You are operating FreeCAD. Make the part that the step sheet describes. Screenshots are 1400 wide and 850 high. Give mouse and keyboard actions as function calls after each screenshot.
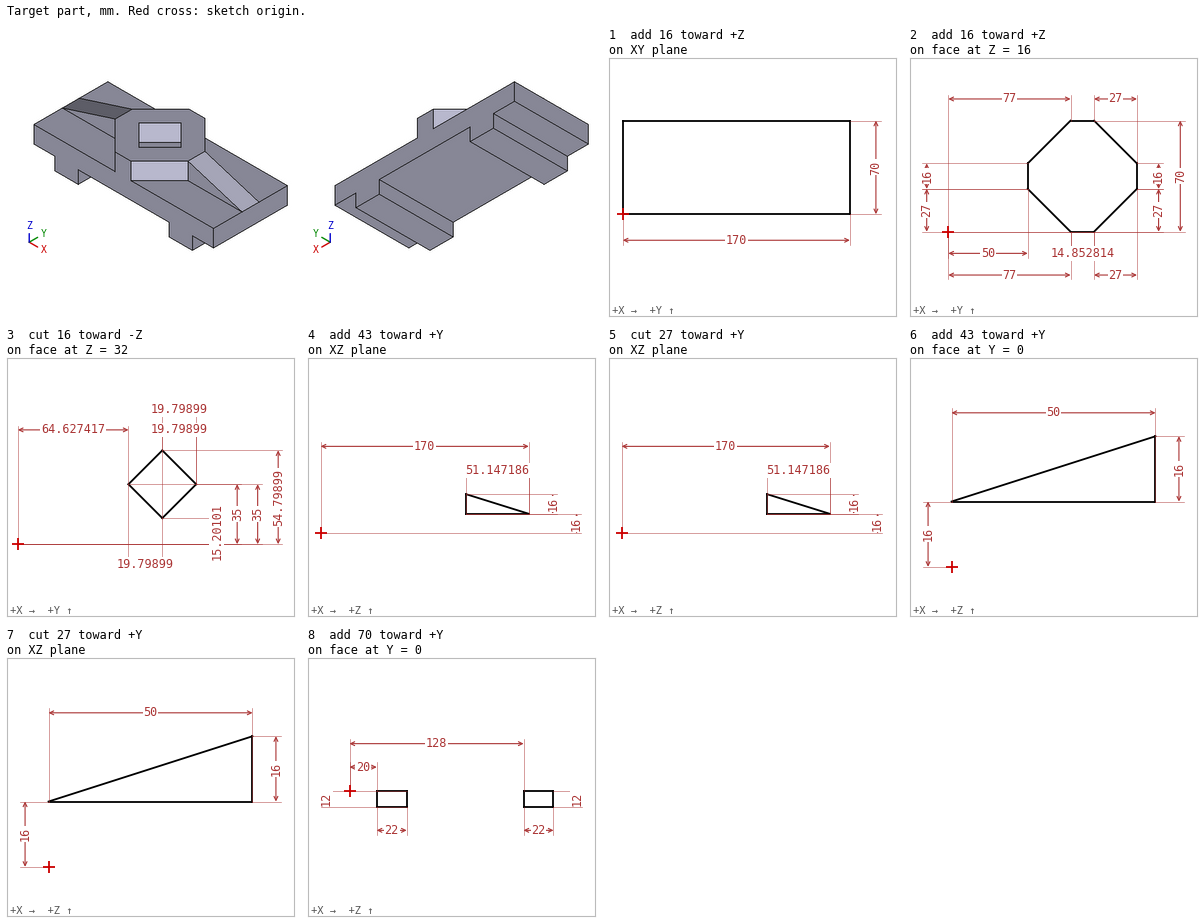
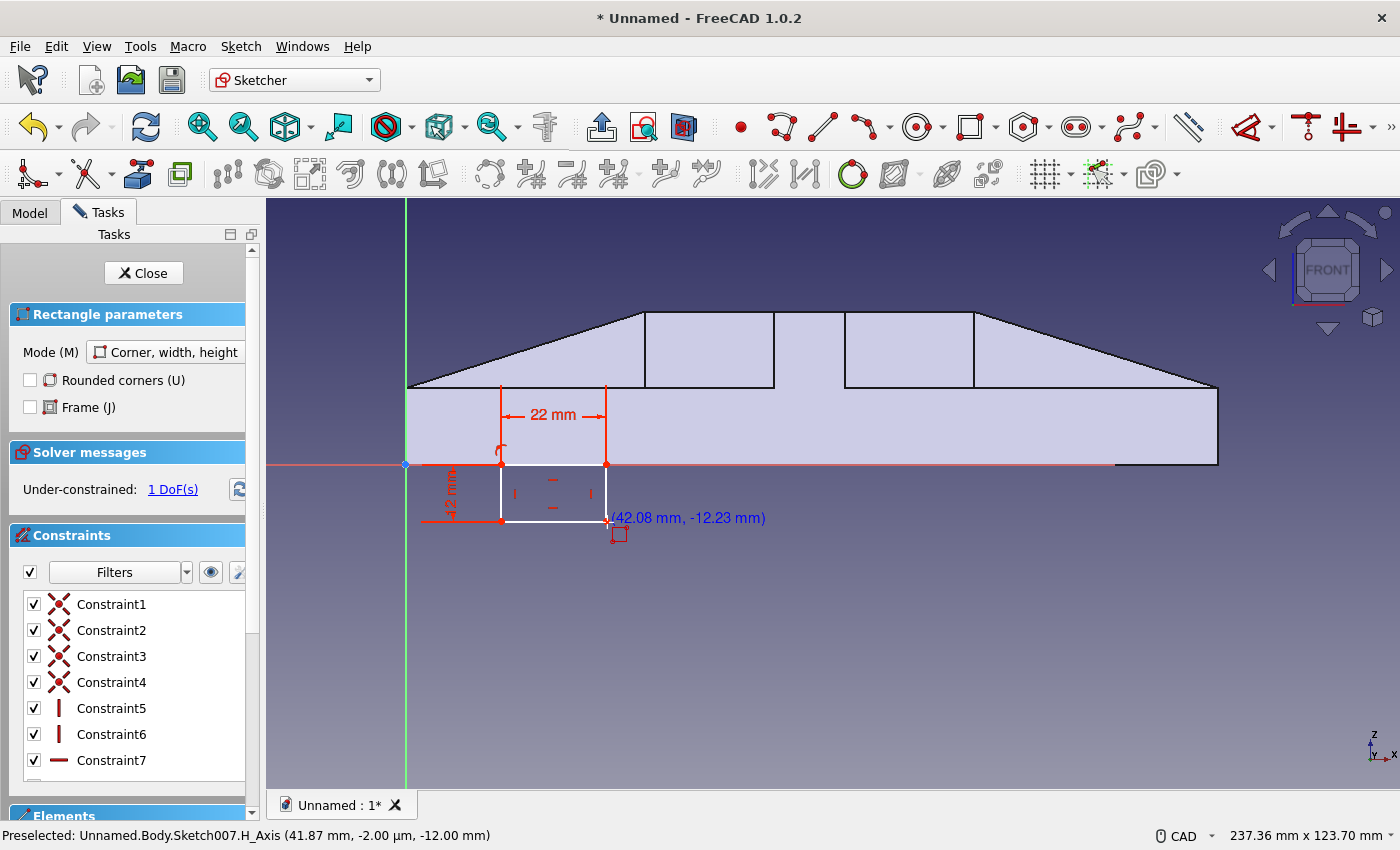
click(1017, 465)
move(1123, 522)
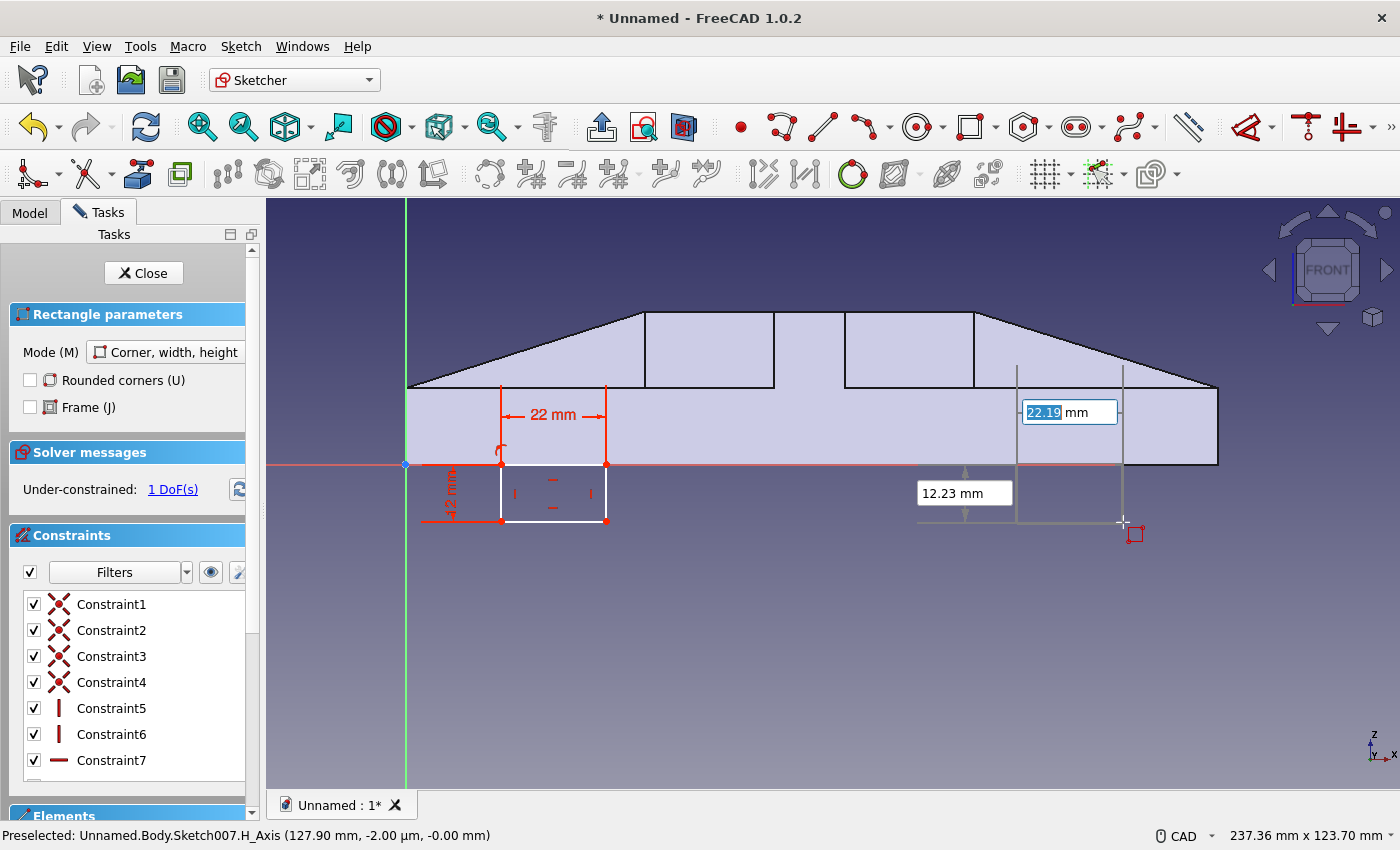
text(22)
key(Tab)
text(12)
key(Return)
key(Escape)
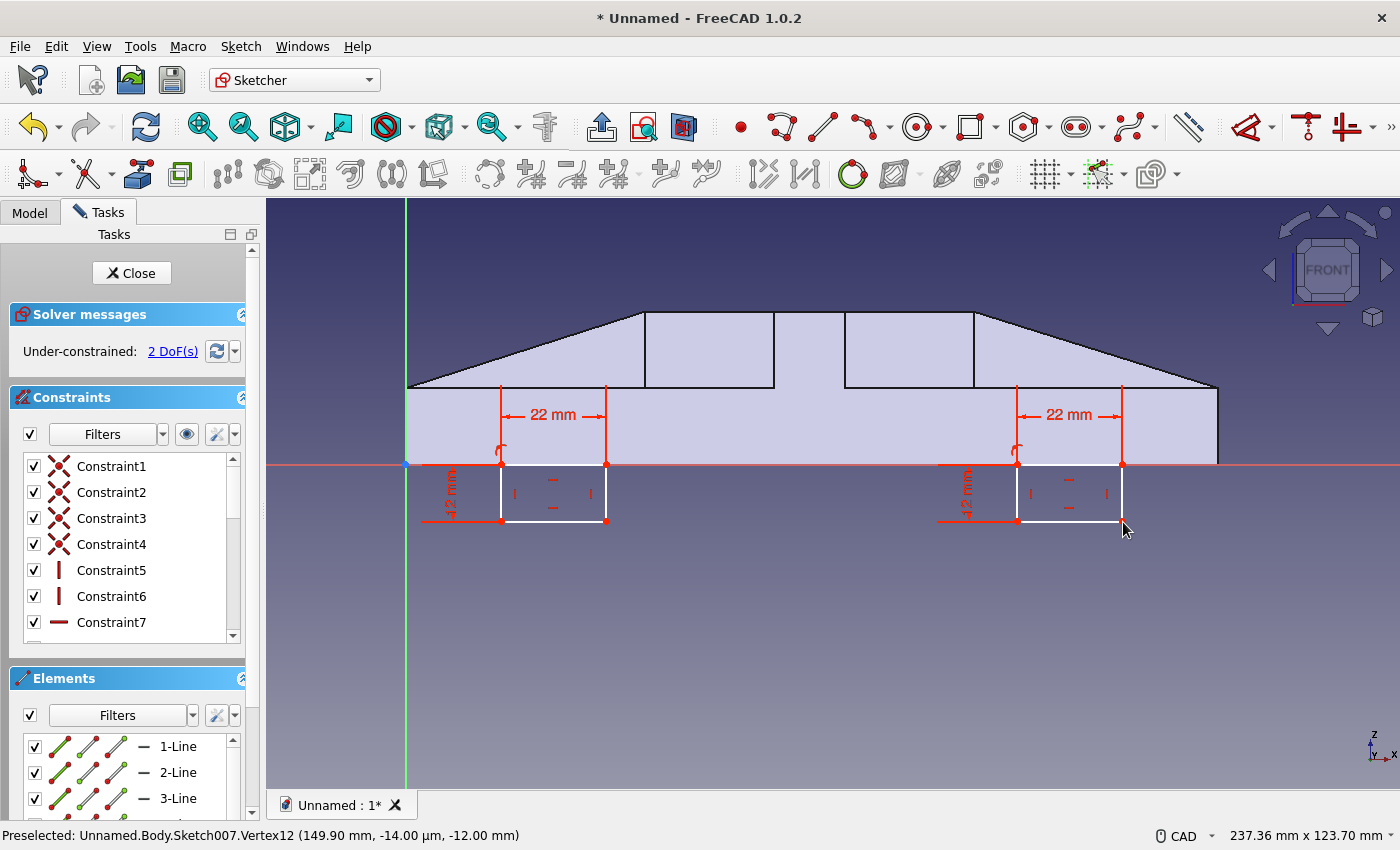
click(1246, 128)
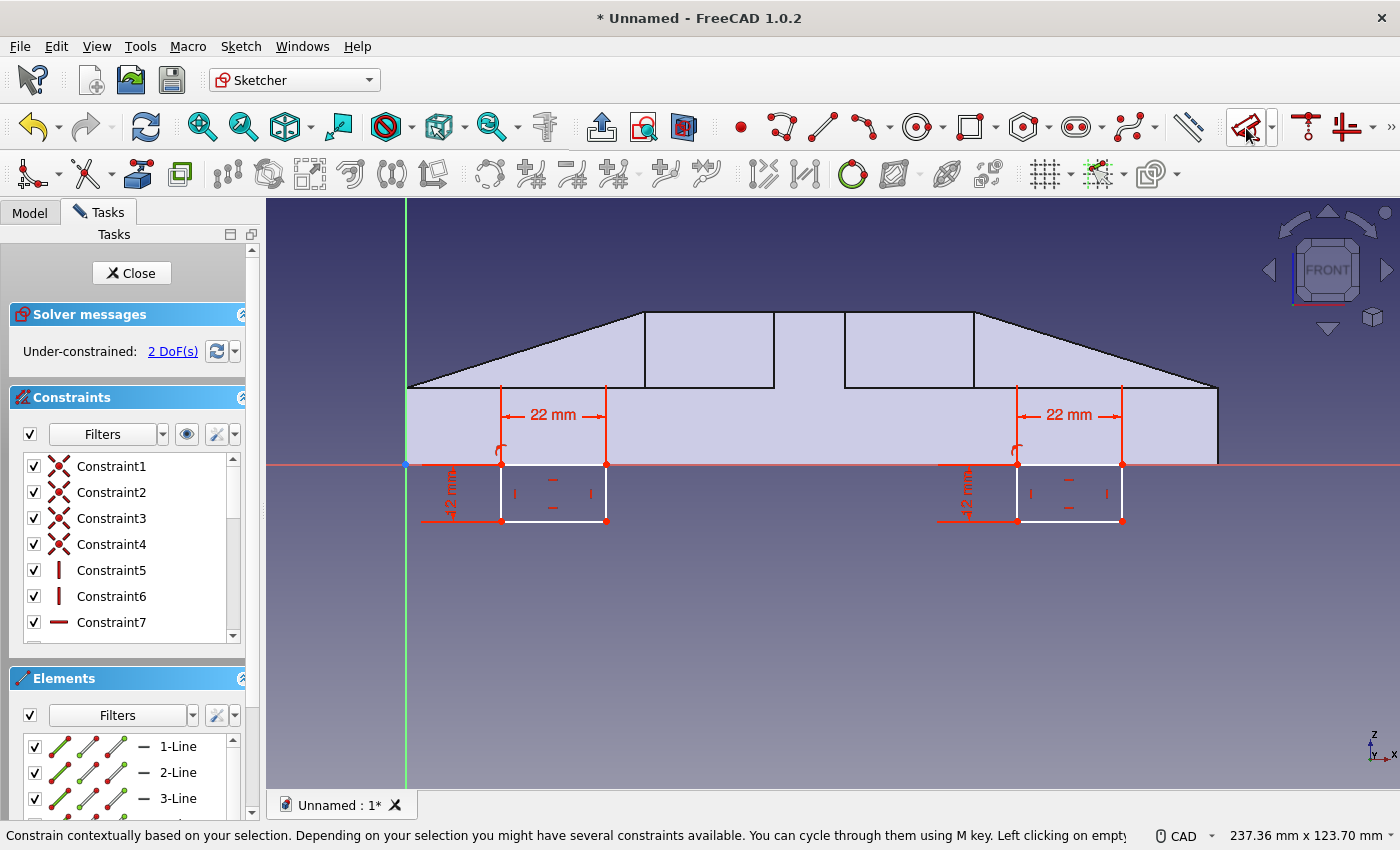
click(501, 465)
click(453, 431)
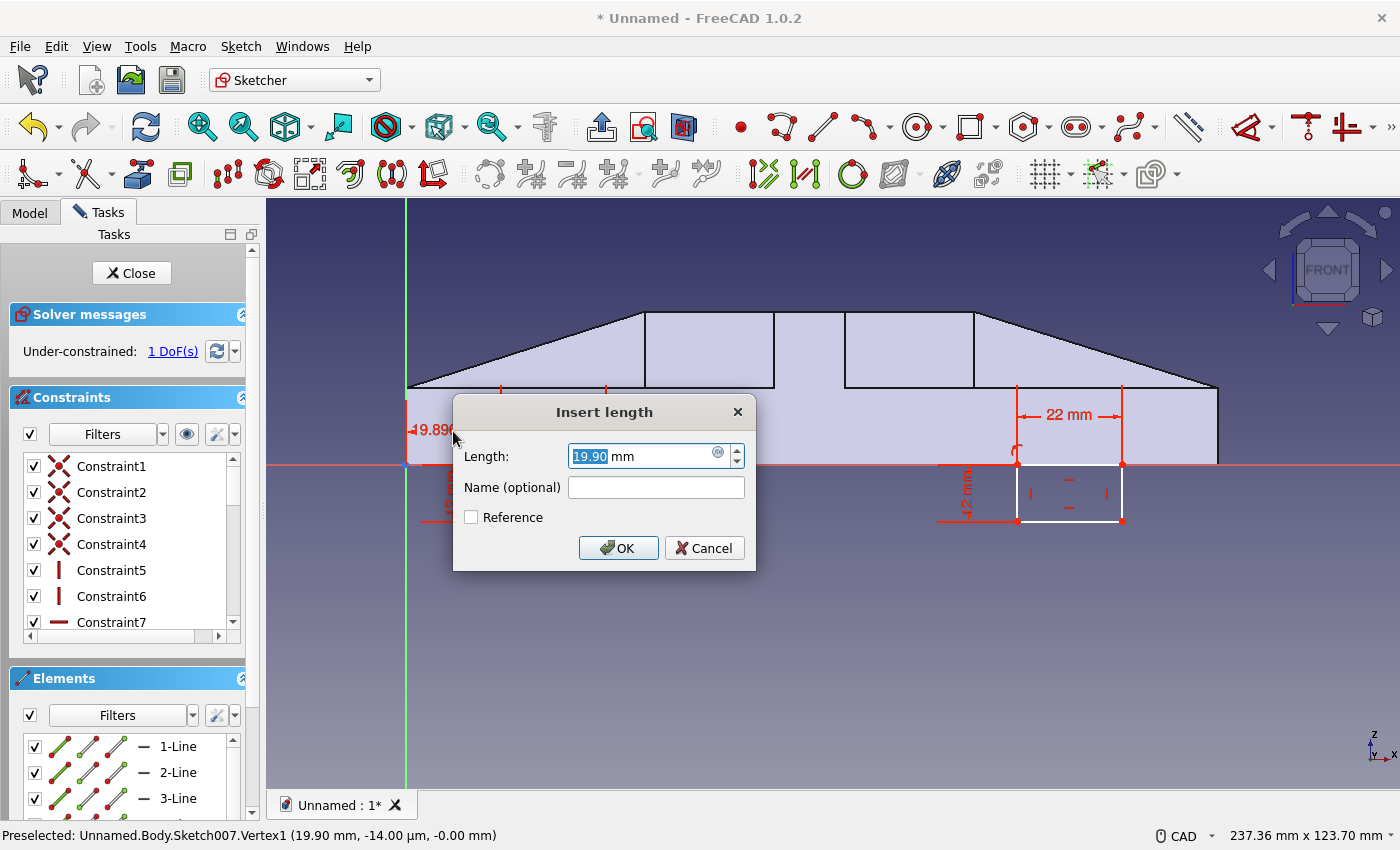
text(20)
key(Return)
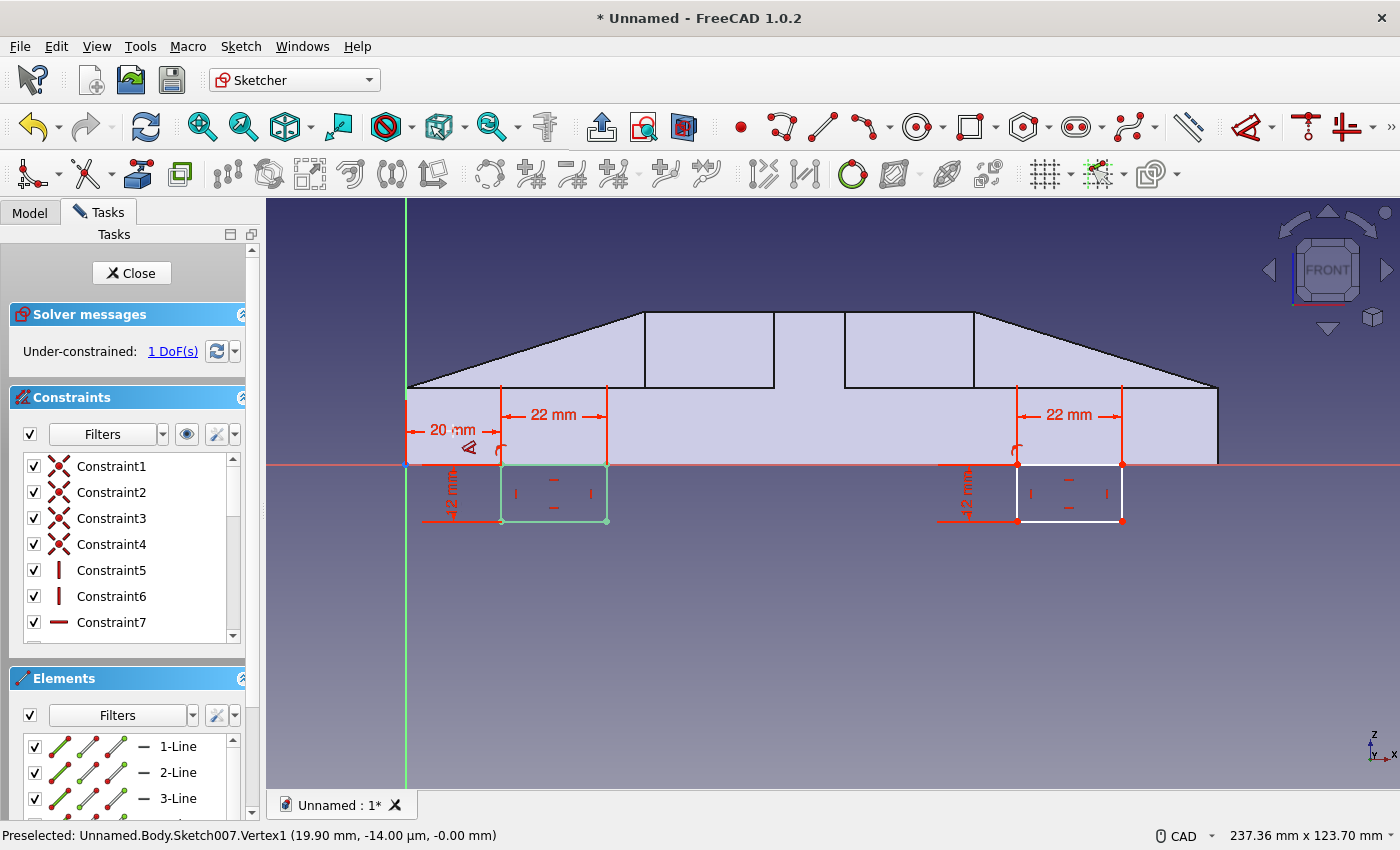
click(1017, 465)
click(711, 431)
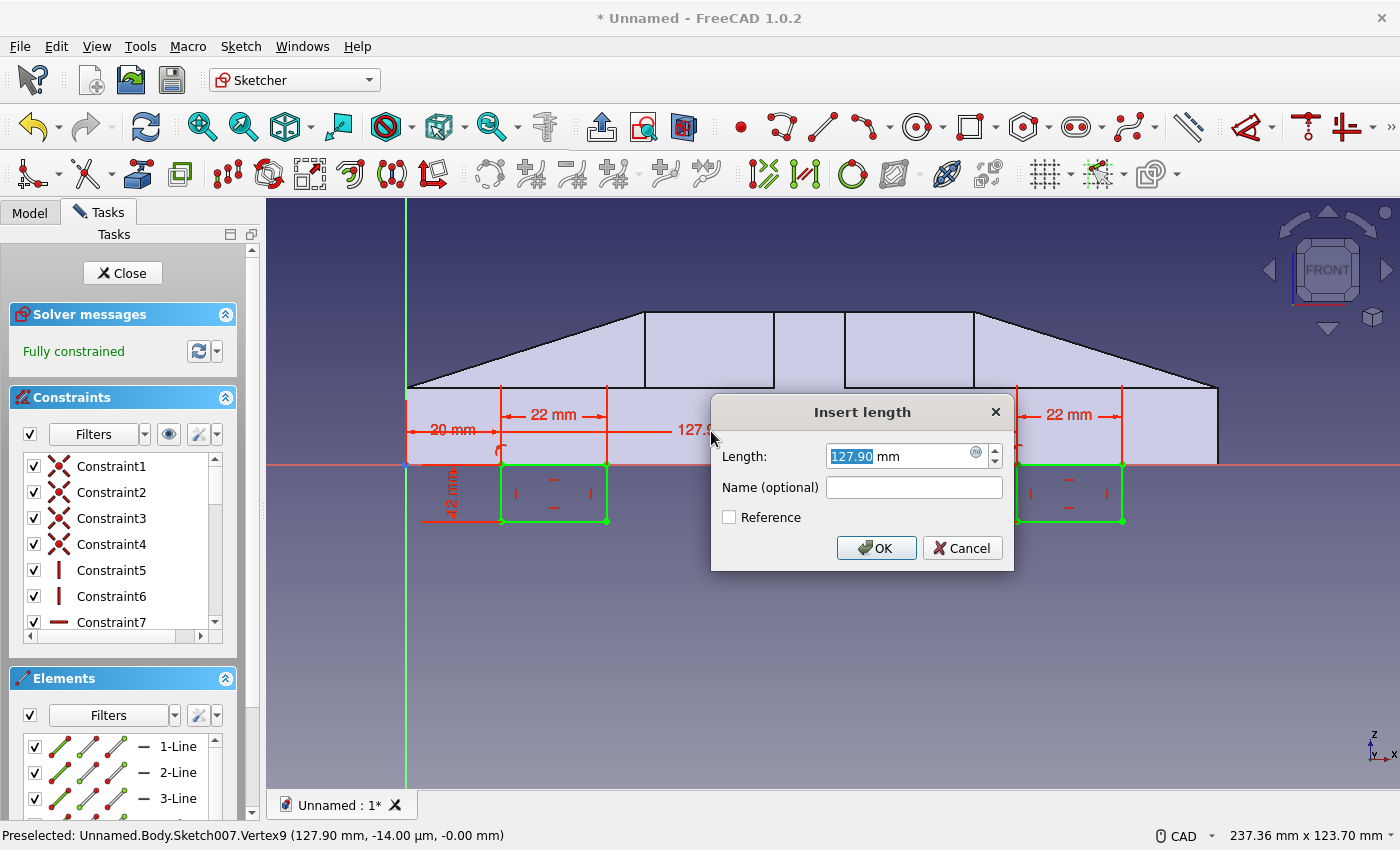
text(128)
key(Return)
key(Escape)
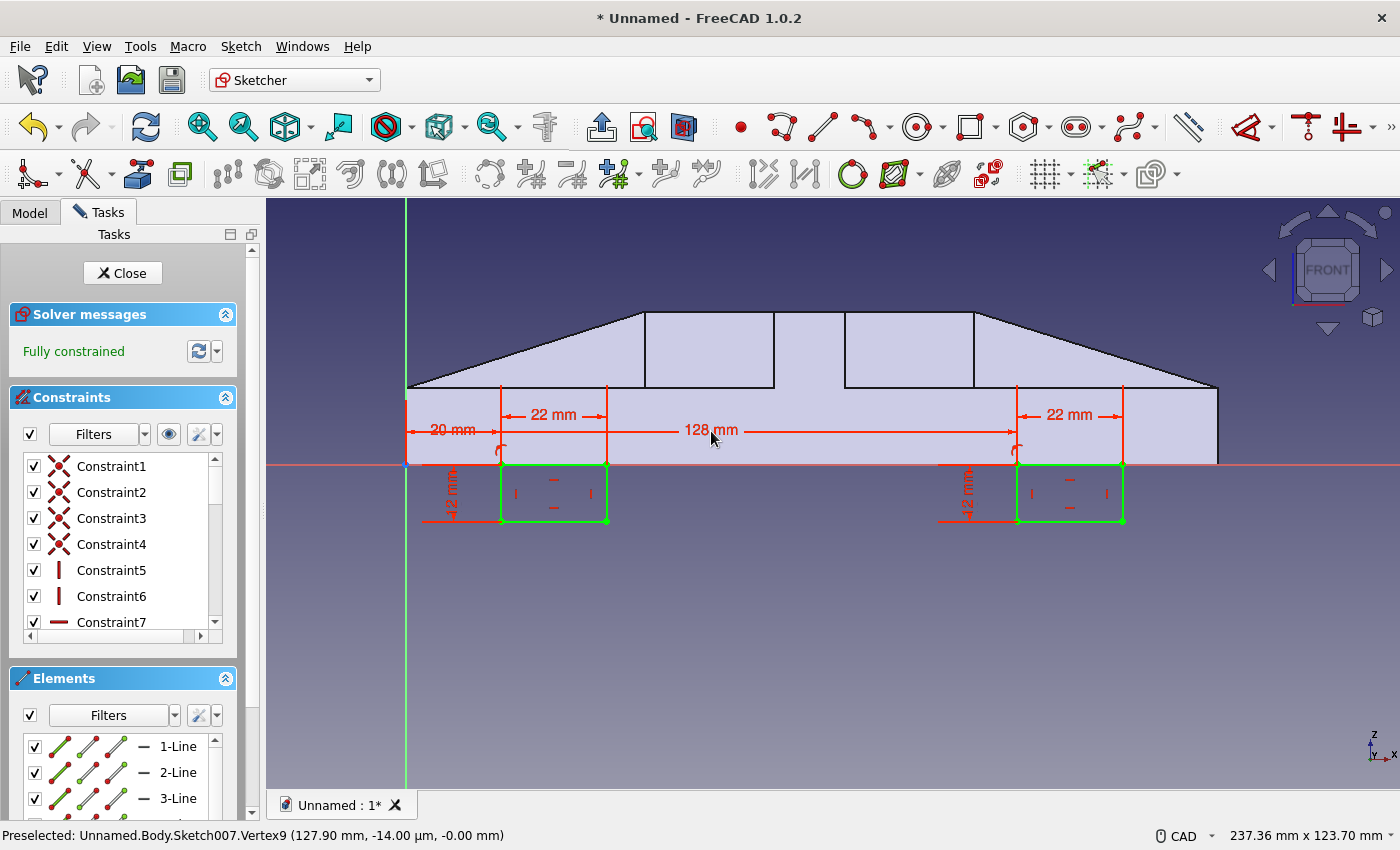
click(123, 273)